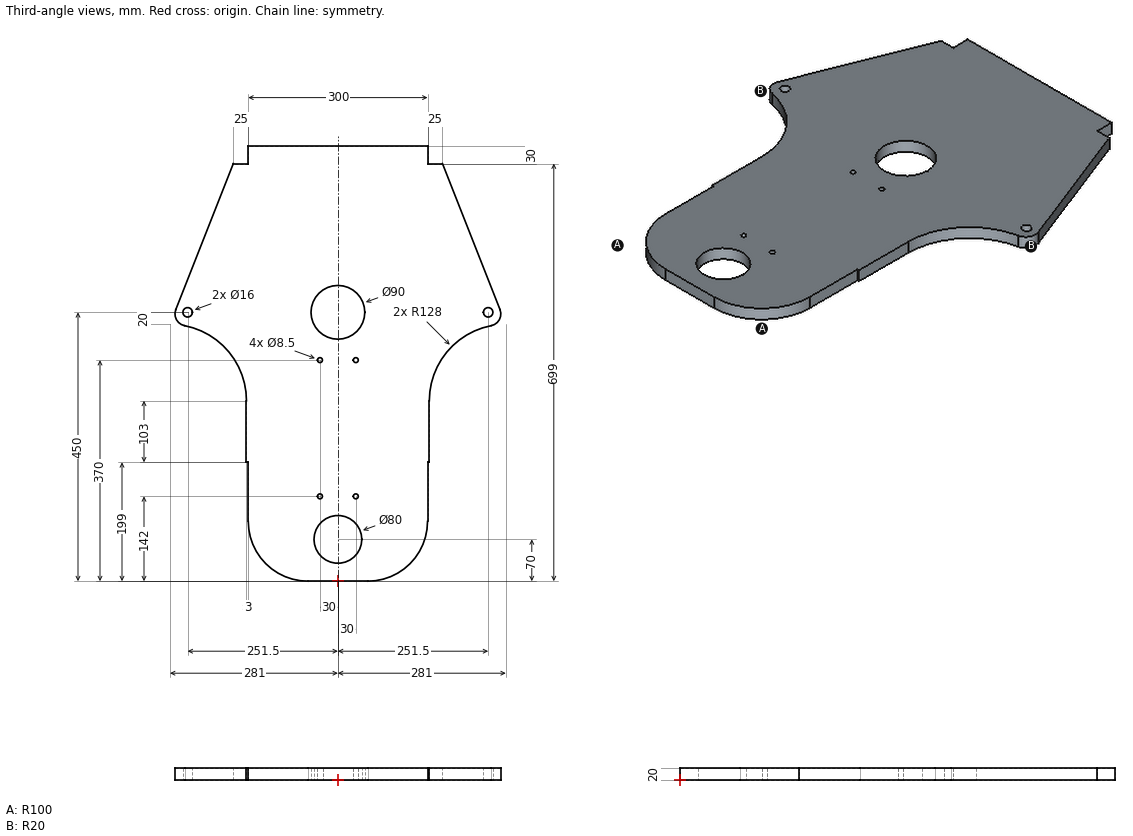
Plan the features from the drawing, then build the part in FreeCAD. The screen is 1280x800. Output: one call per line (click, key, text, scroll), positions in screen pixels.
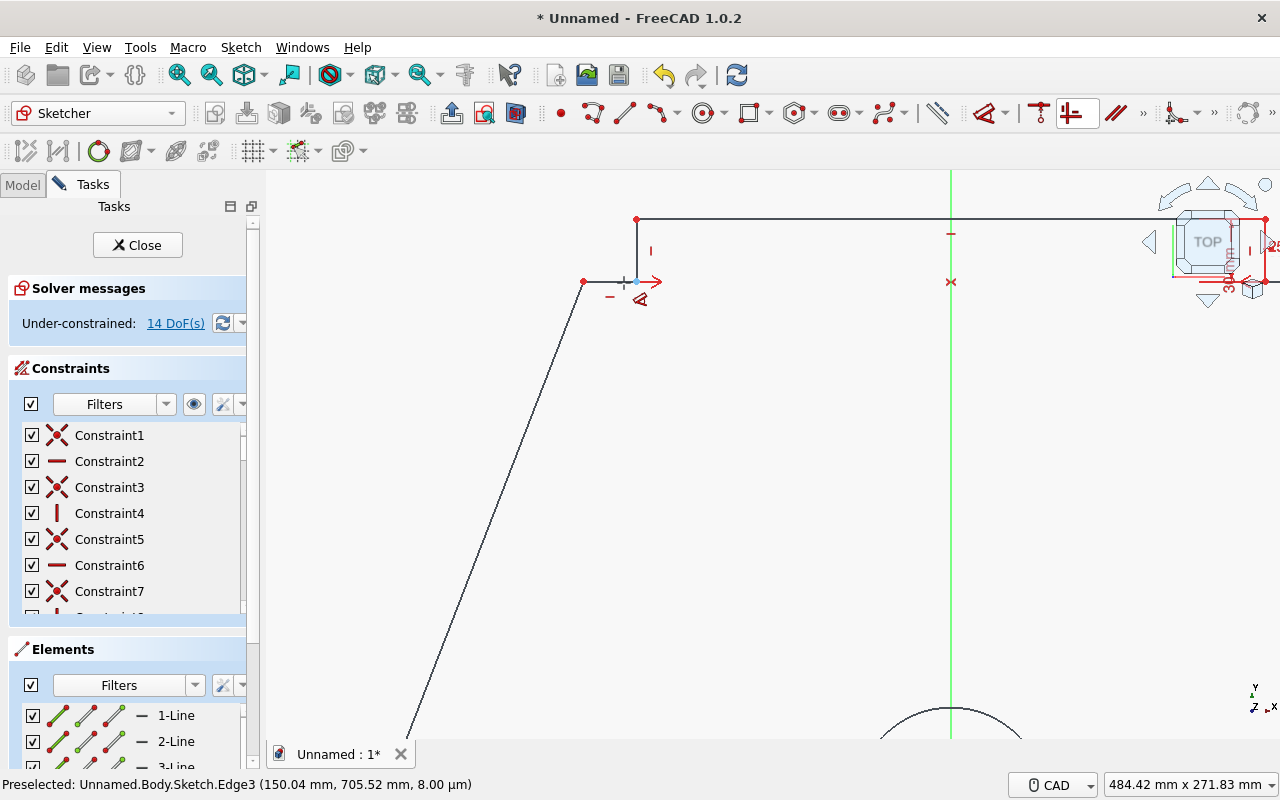
click(621, 282)
click(610, 248)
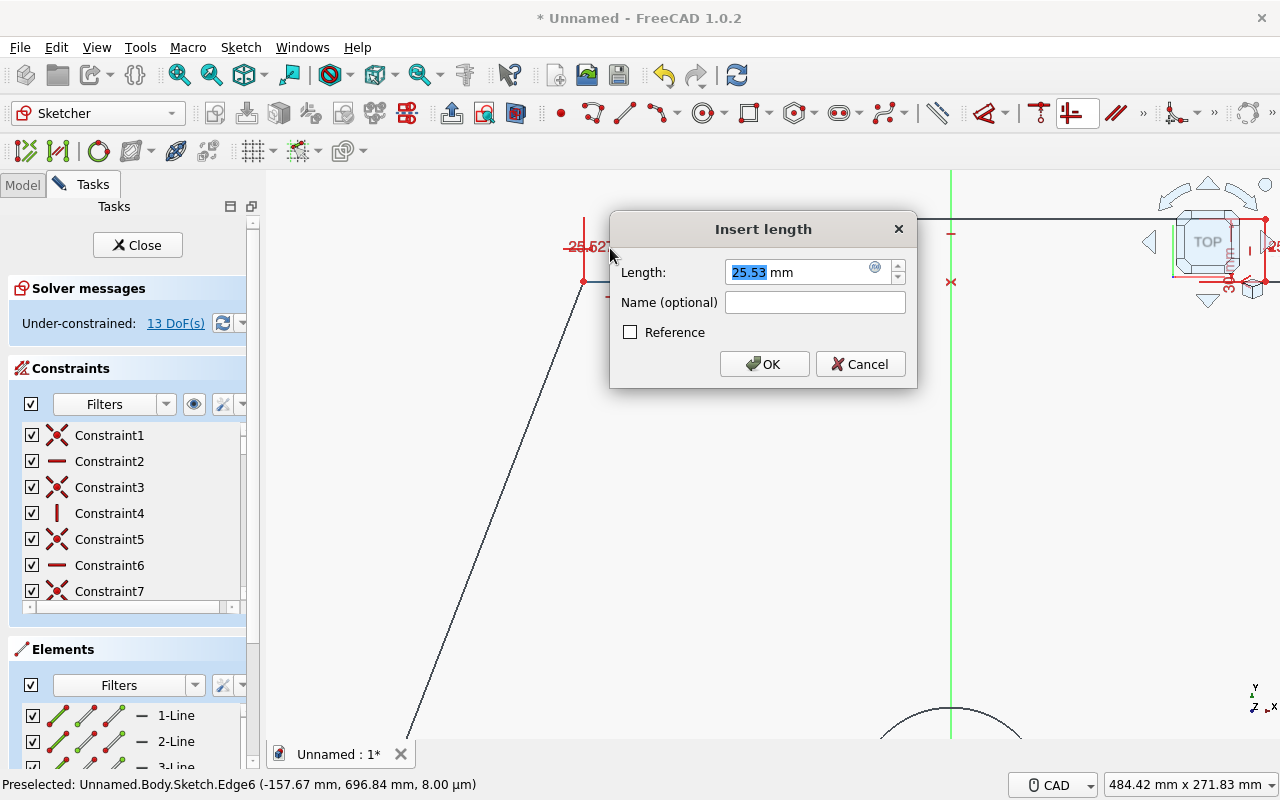
text(25)
key(Return)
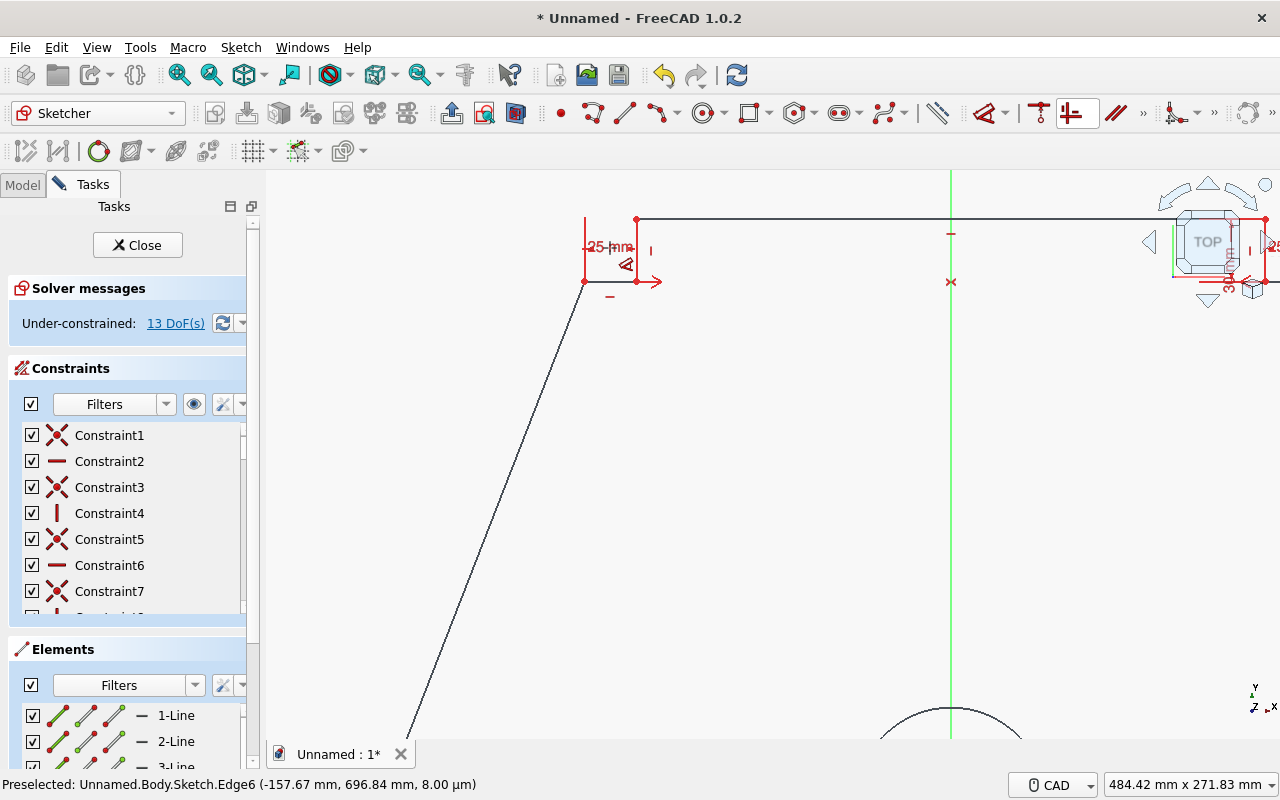
scroll(624, 283, down, 7)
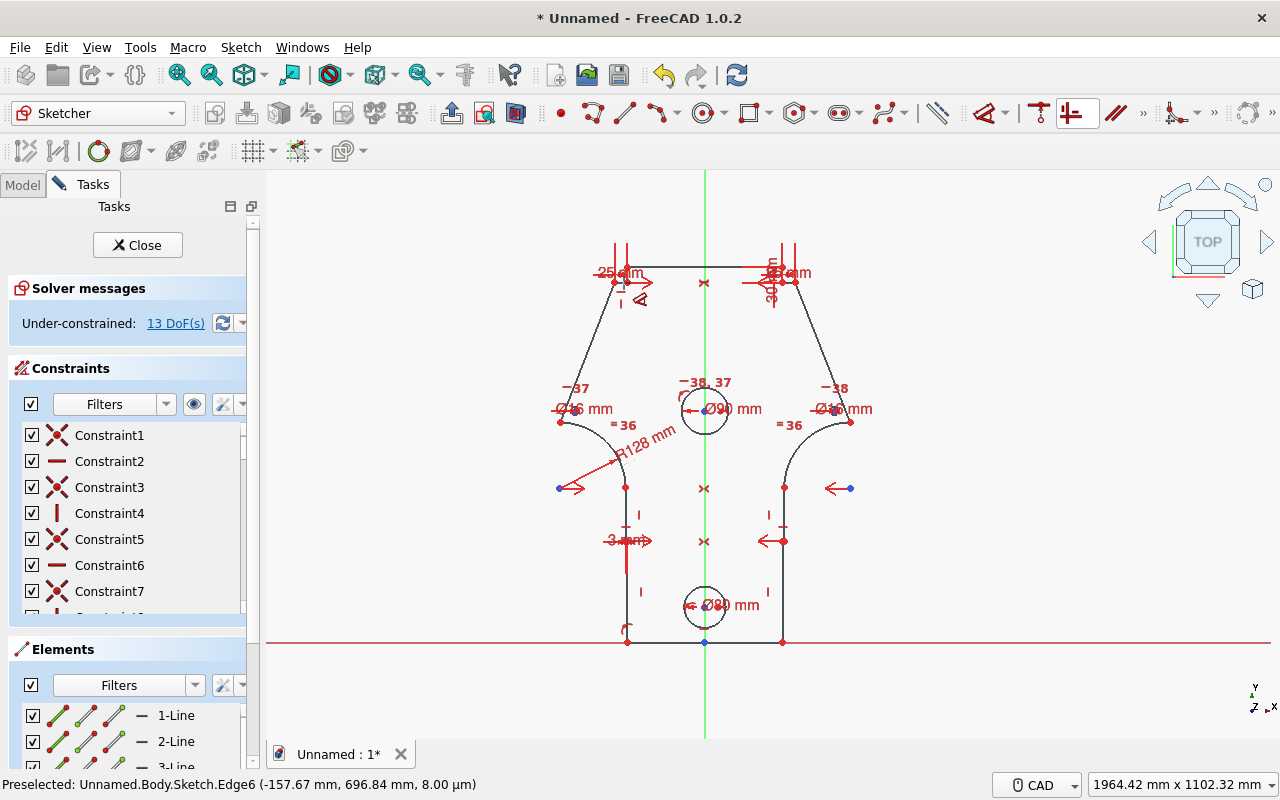
click(705, 607)
click(739, 625)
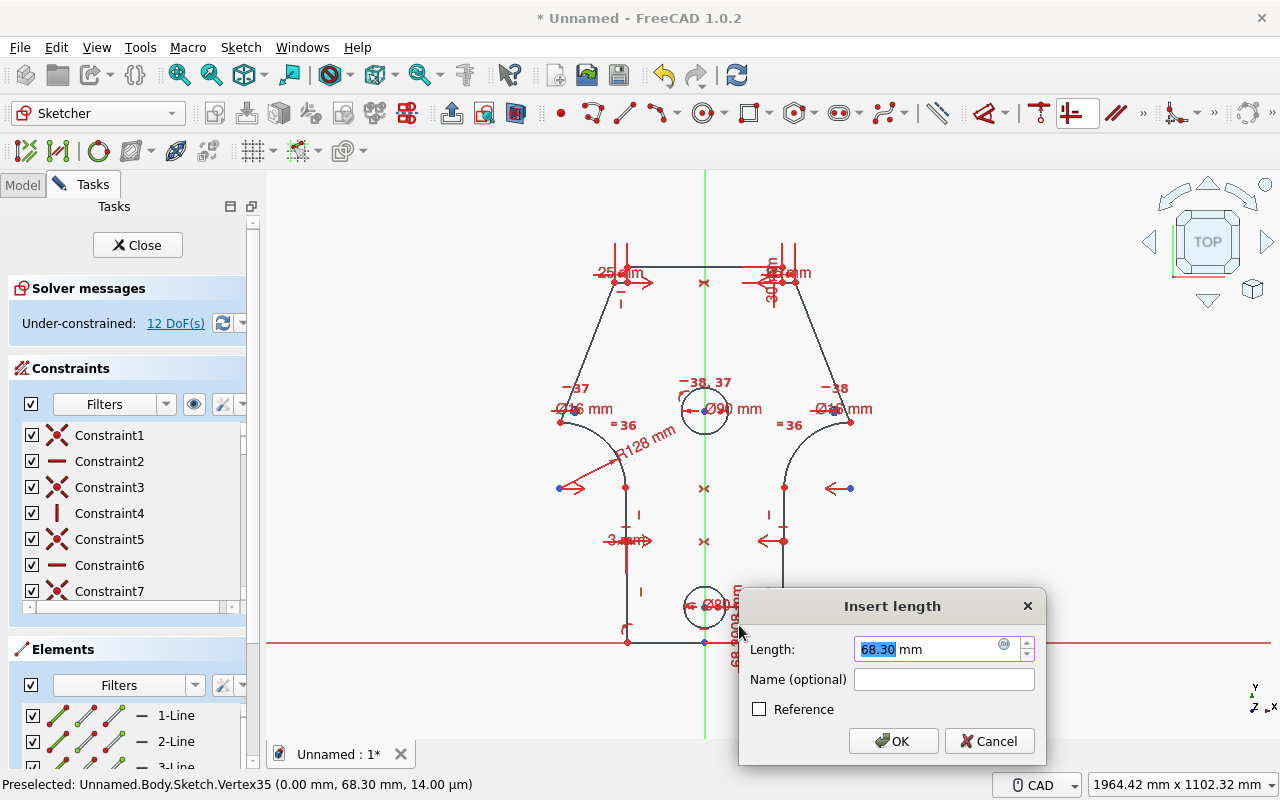
text(70)
key(Return)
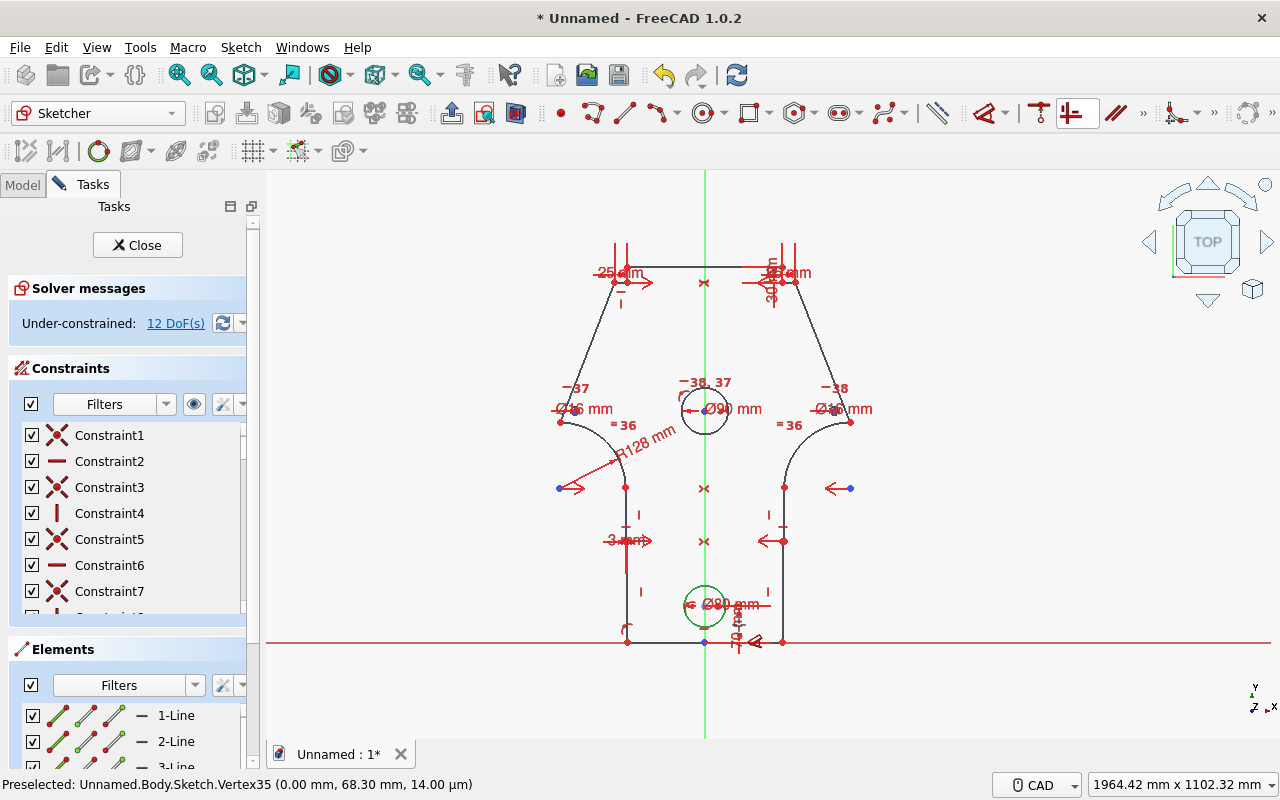
click(736, 267)
click(669, 233)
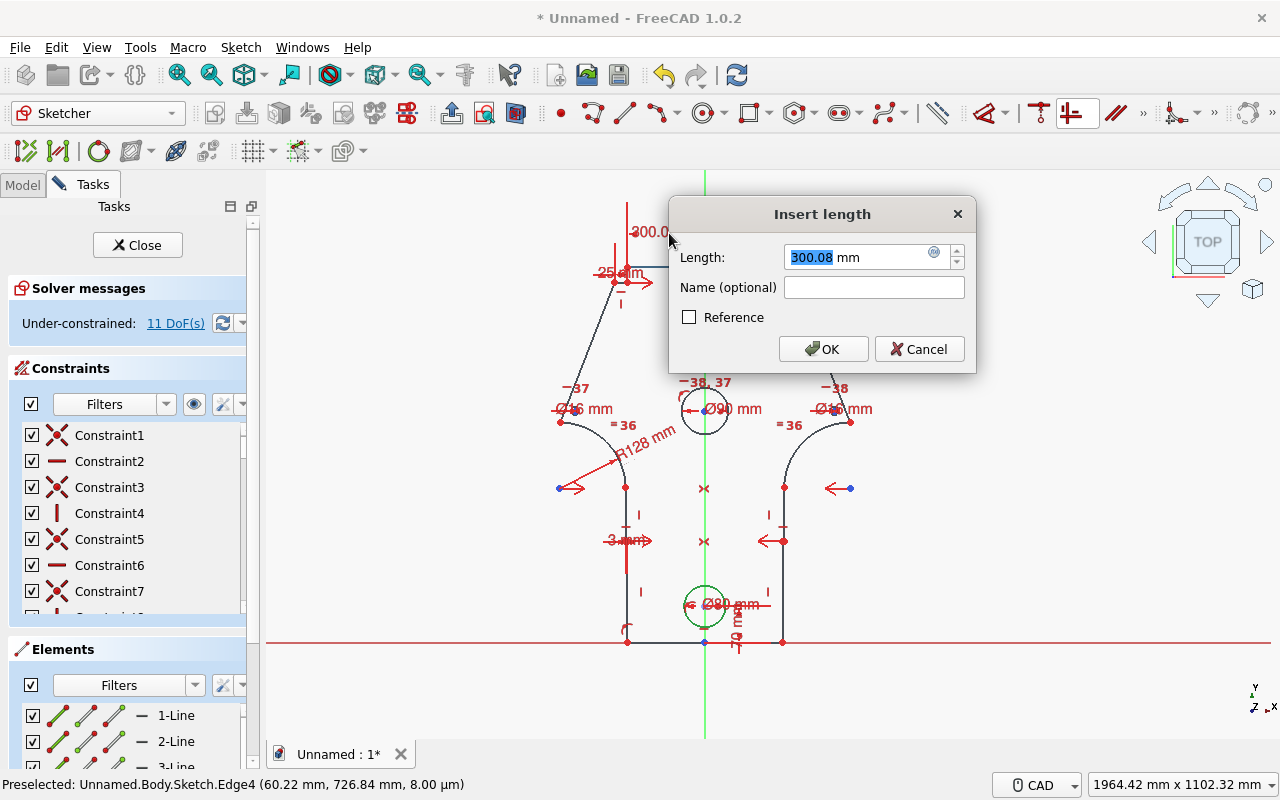
text(300)
key(Return)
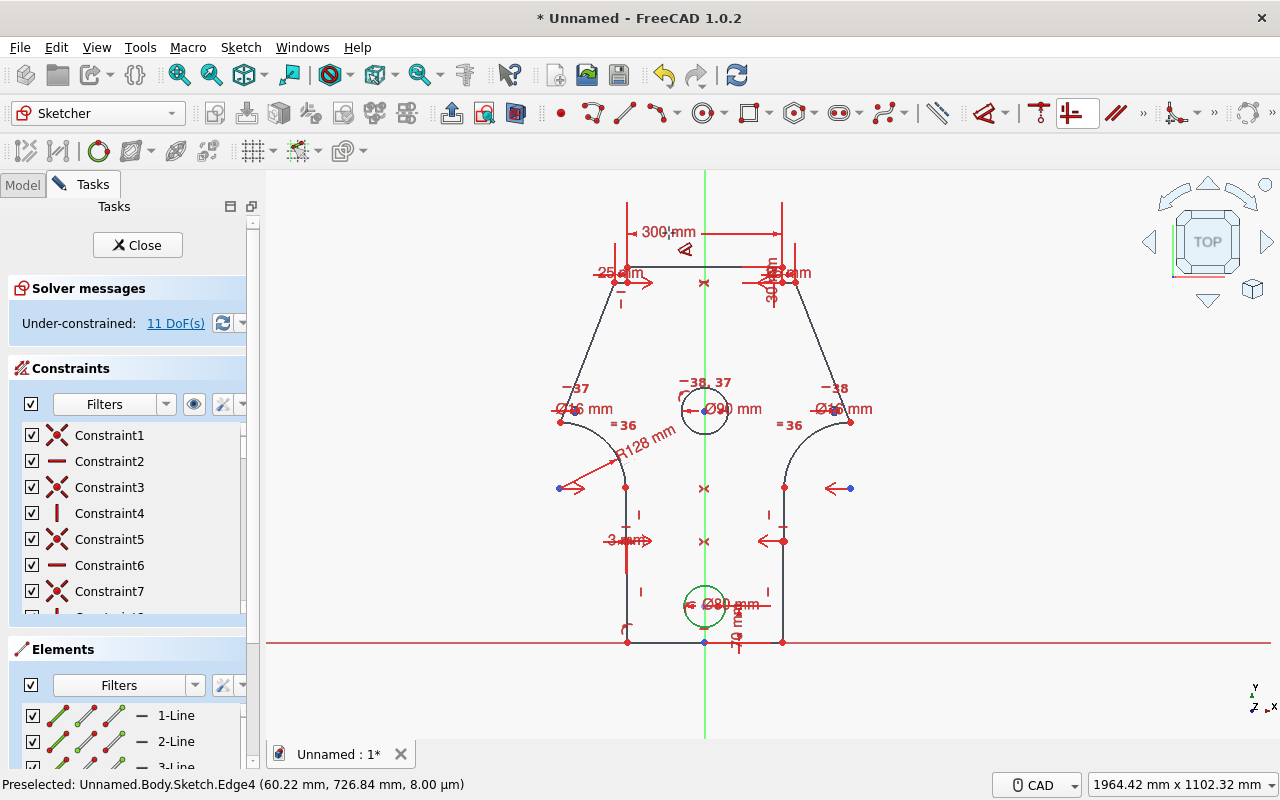
click(626, 504)
click(592, 514)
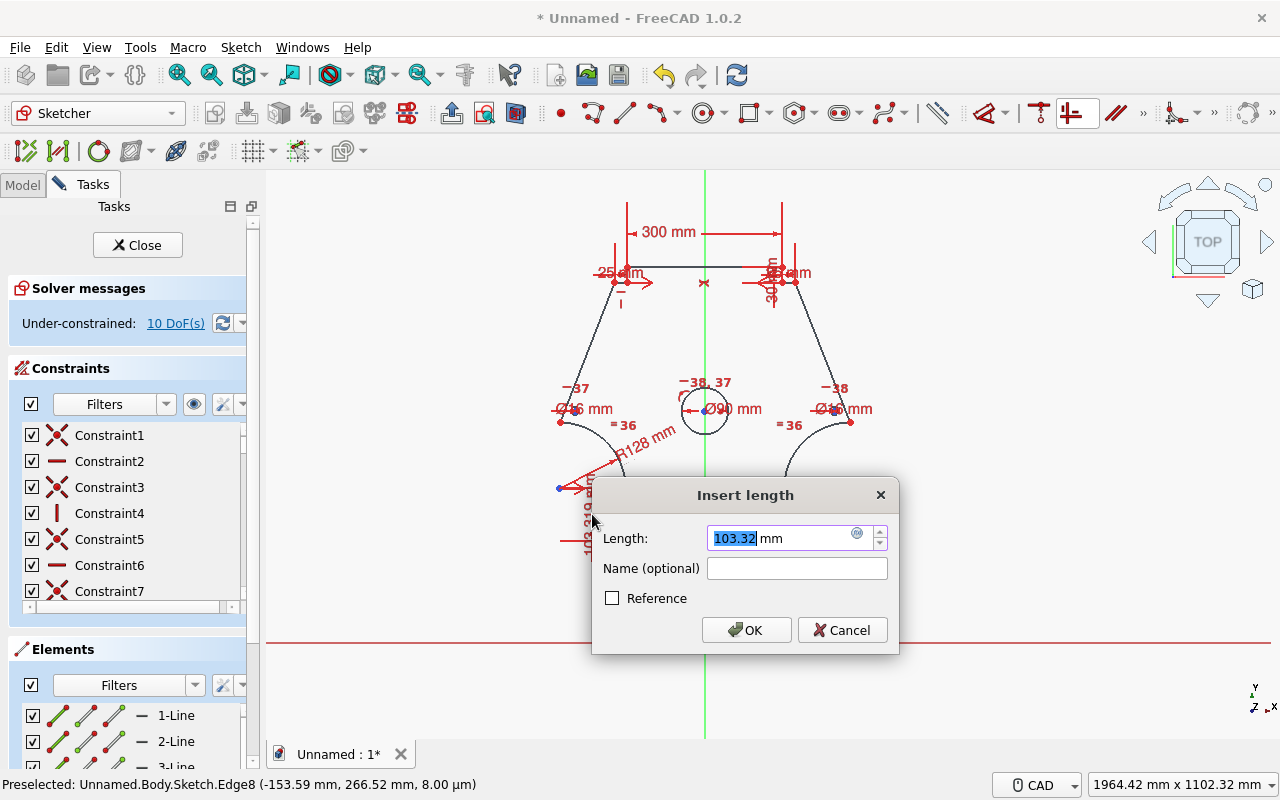
text(103)
key(Return)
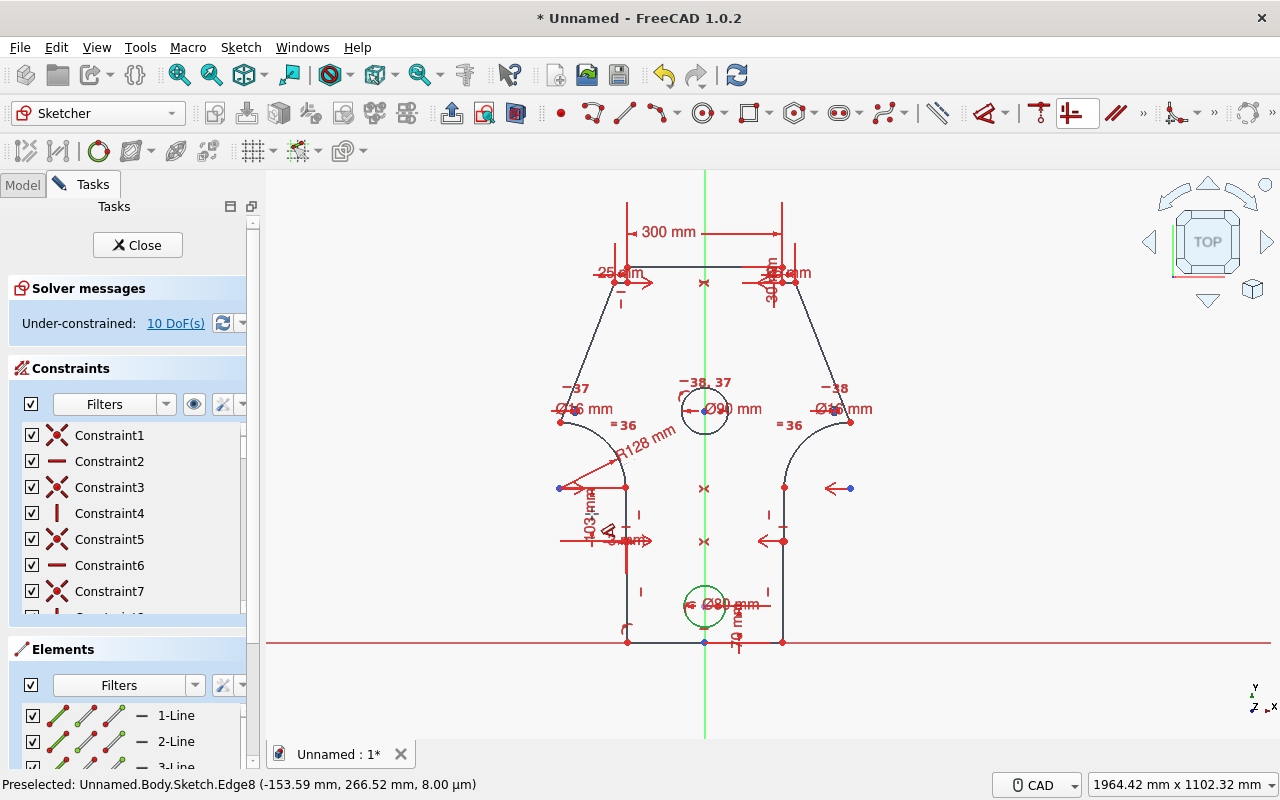
click(627, 571)
click(593, 592)